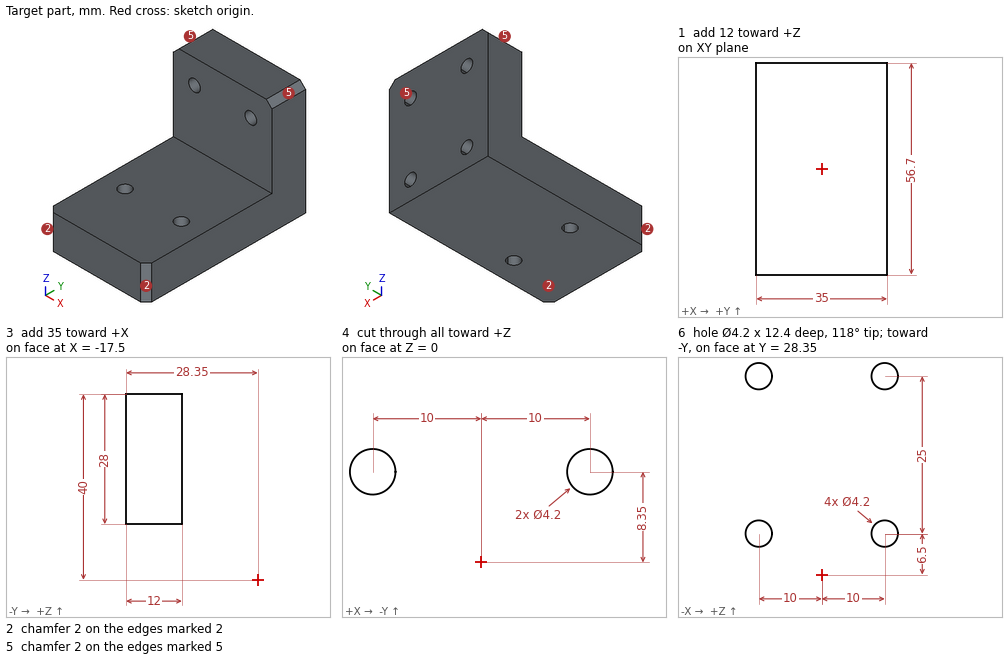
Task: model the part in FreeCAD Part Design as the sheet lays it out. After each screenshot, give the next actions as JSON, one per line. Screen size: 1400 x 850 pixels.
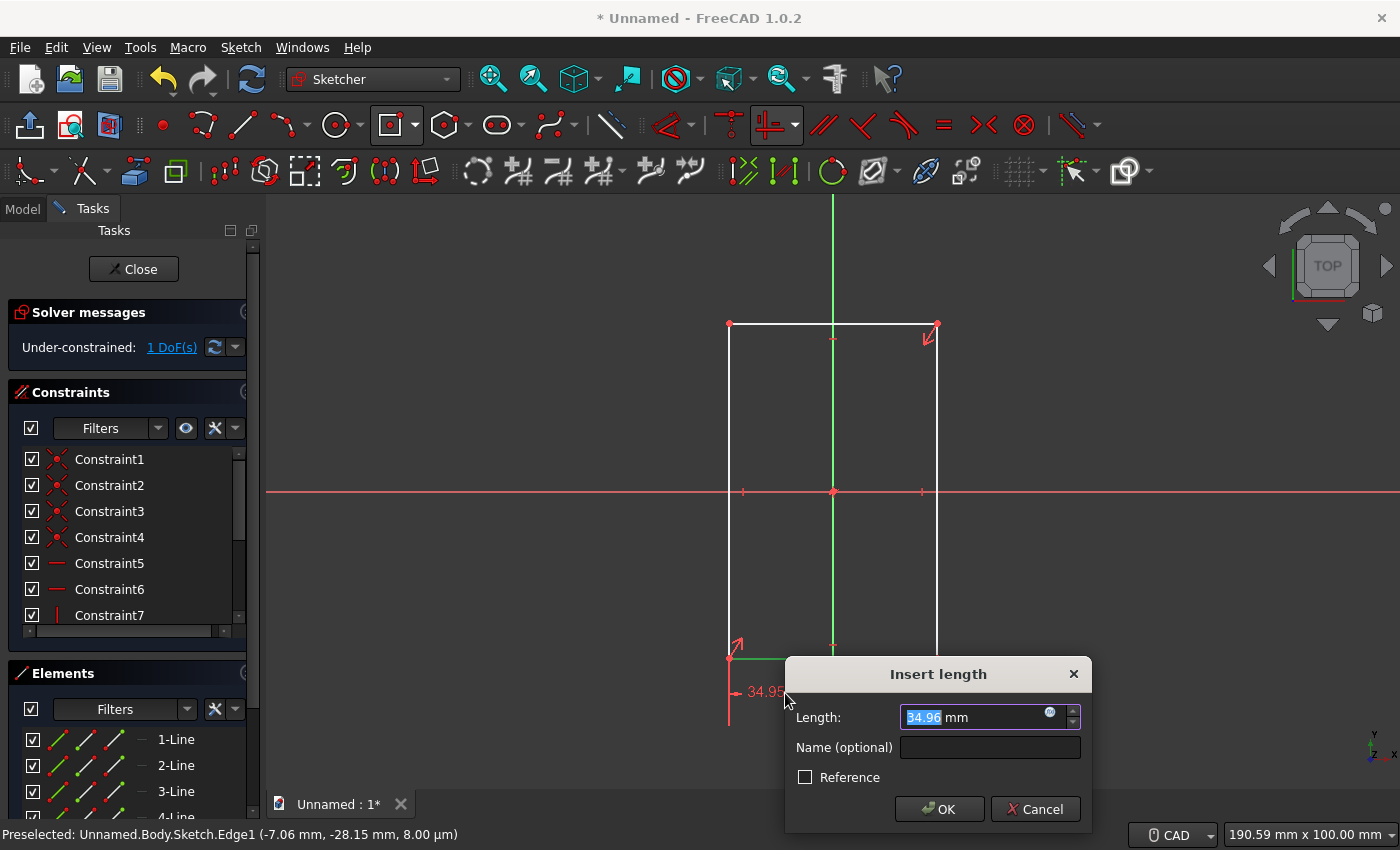
{"action": "type", "text": "35"}
{"action": "key", "text": "Return"}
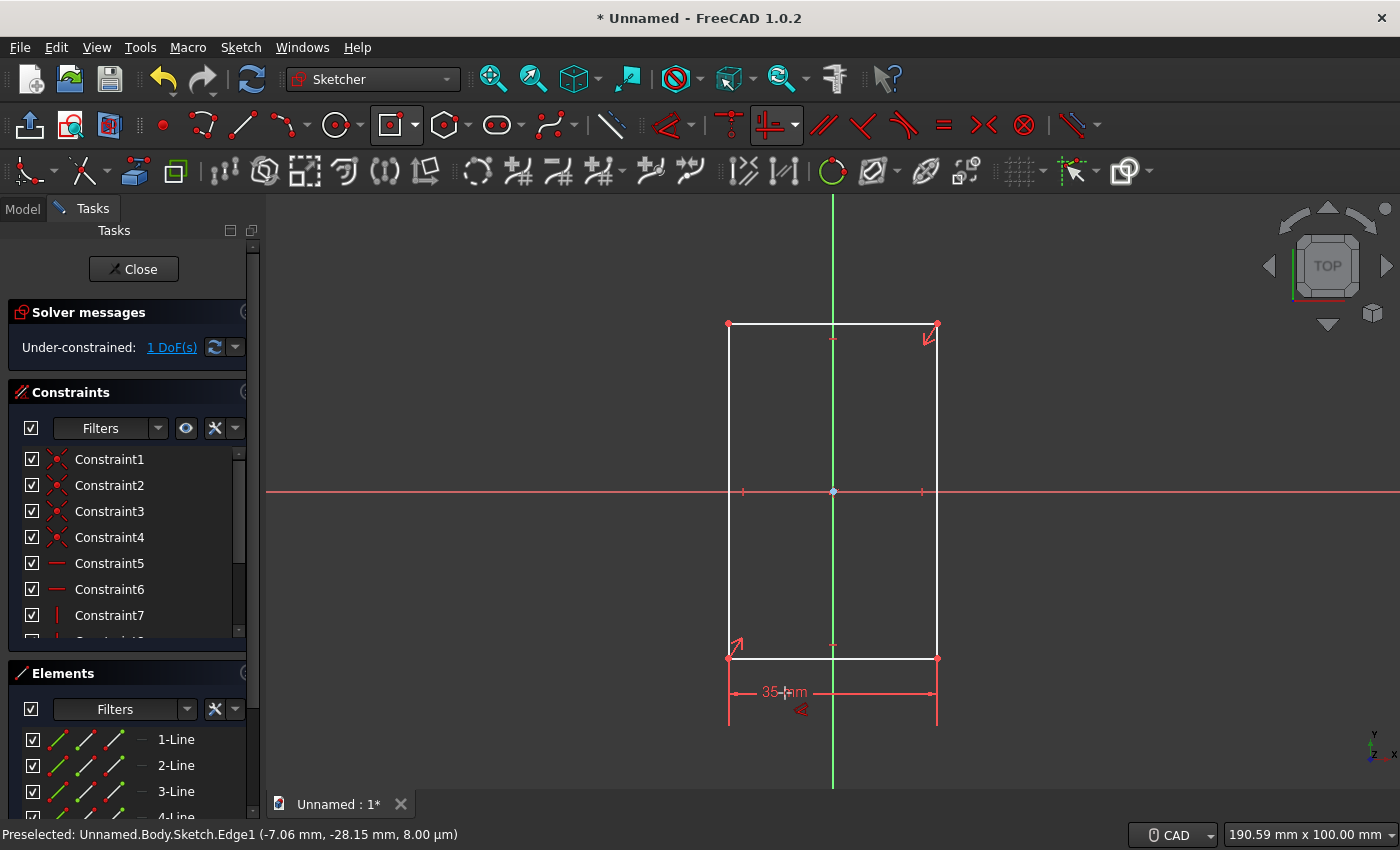
{"action": "left_click", "coordinate": [937, 559]}
{"action": "left_click", "coordinate": [971, 414]}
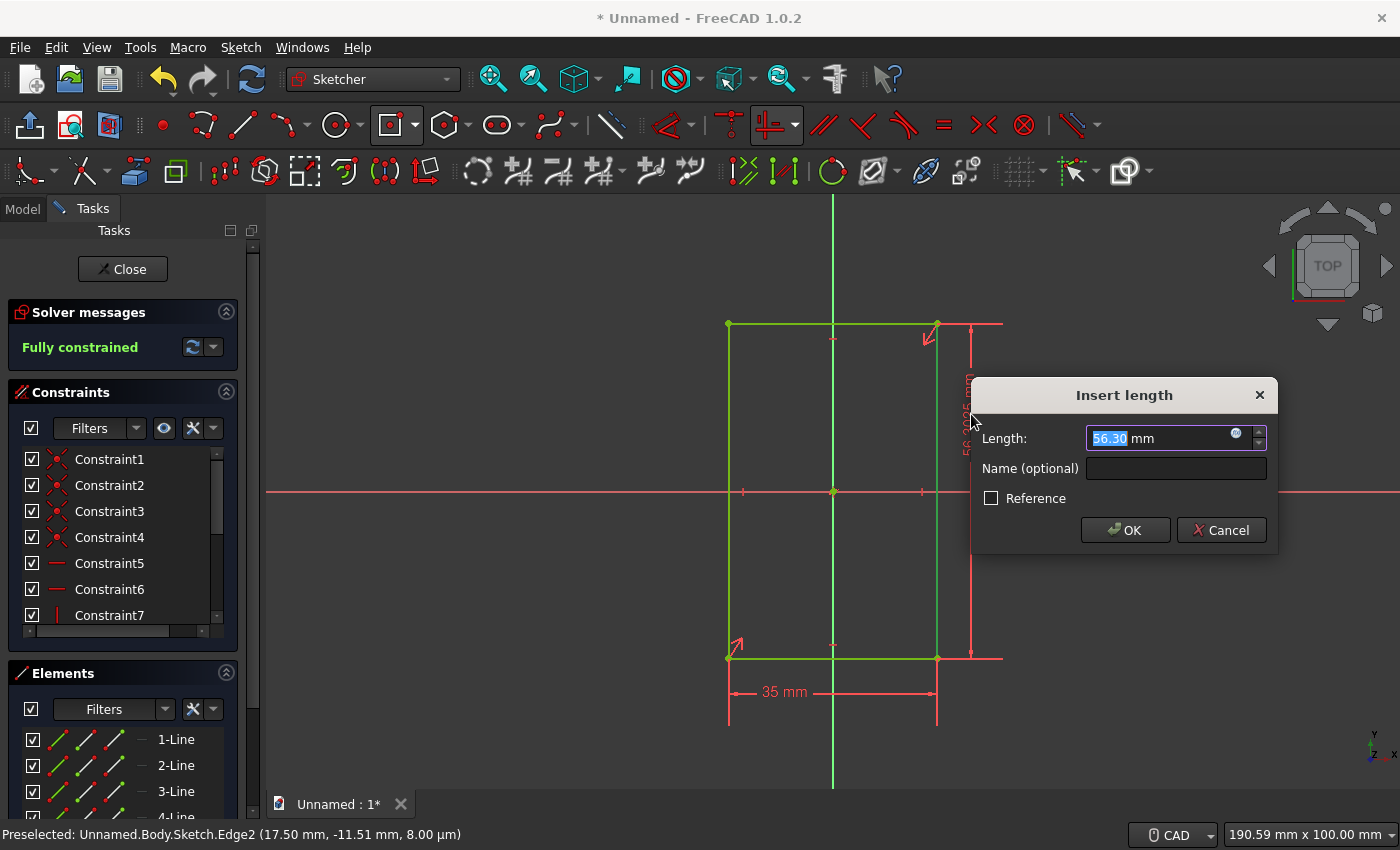
{"action": "type", "text": "56.7"}
{"action": "key", "text": "Return"}
{"action": "key", "text": "Escape"}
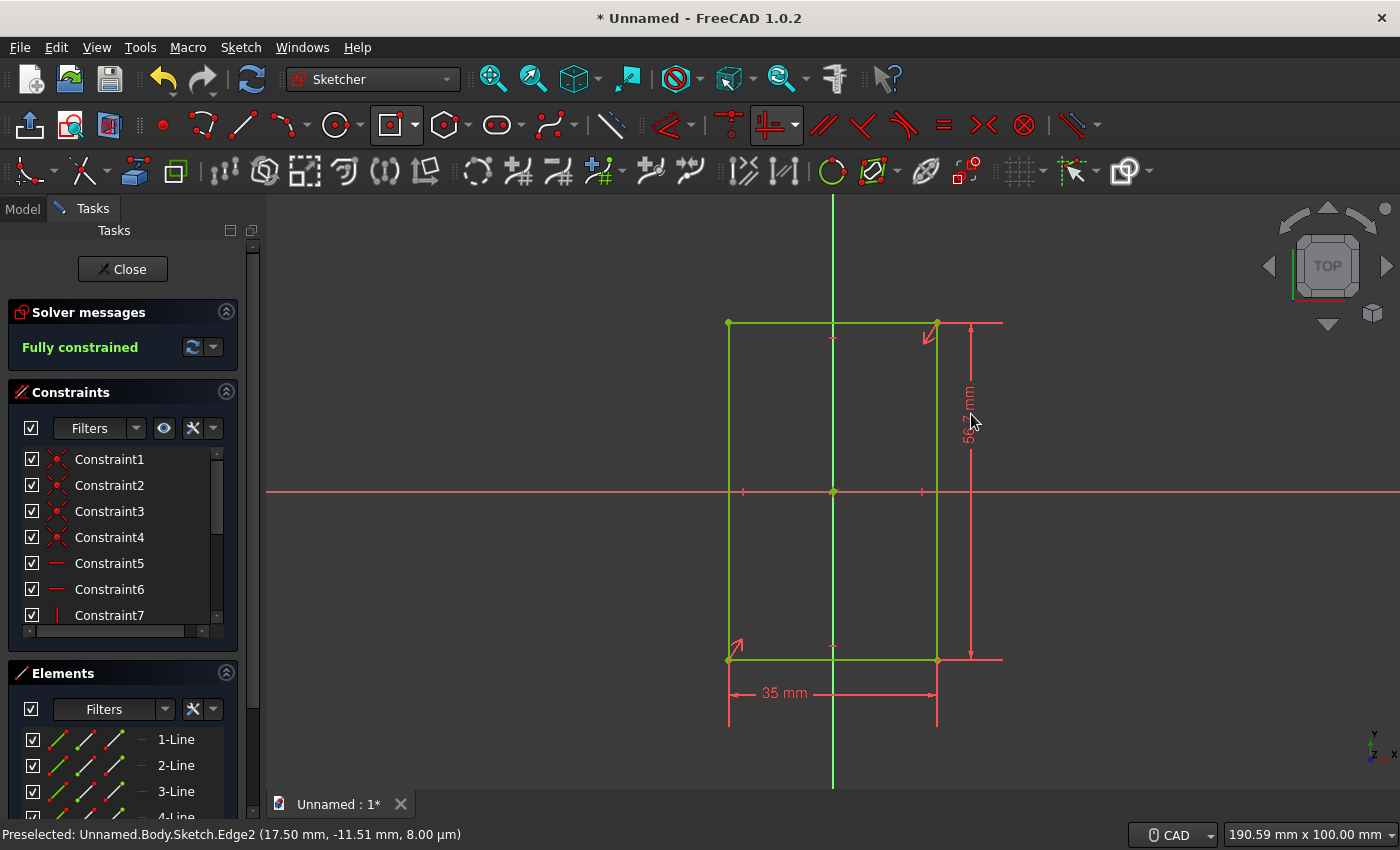
{"action": "left_click", "coordinate": [123, 269]}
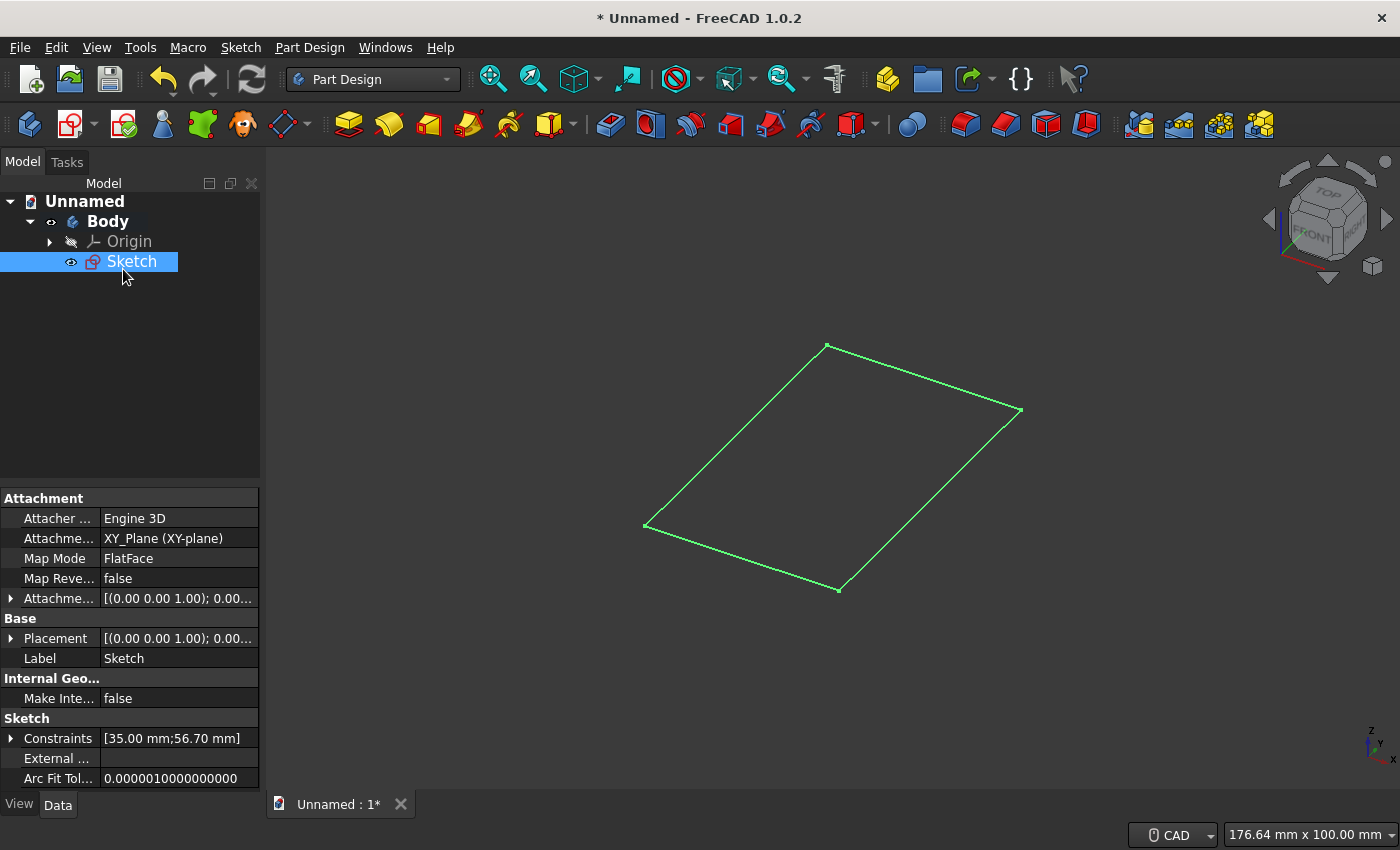
{"action": "left_click", "coordinate": [350, 124]}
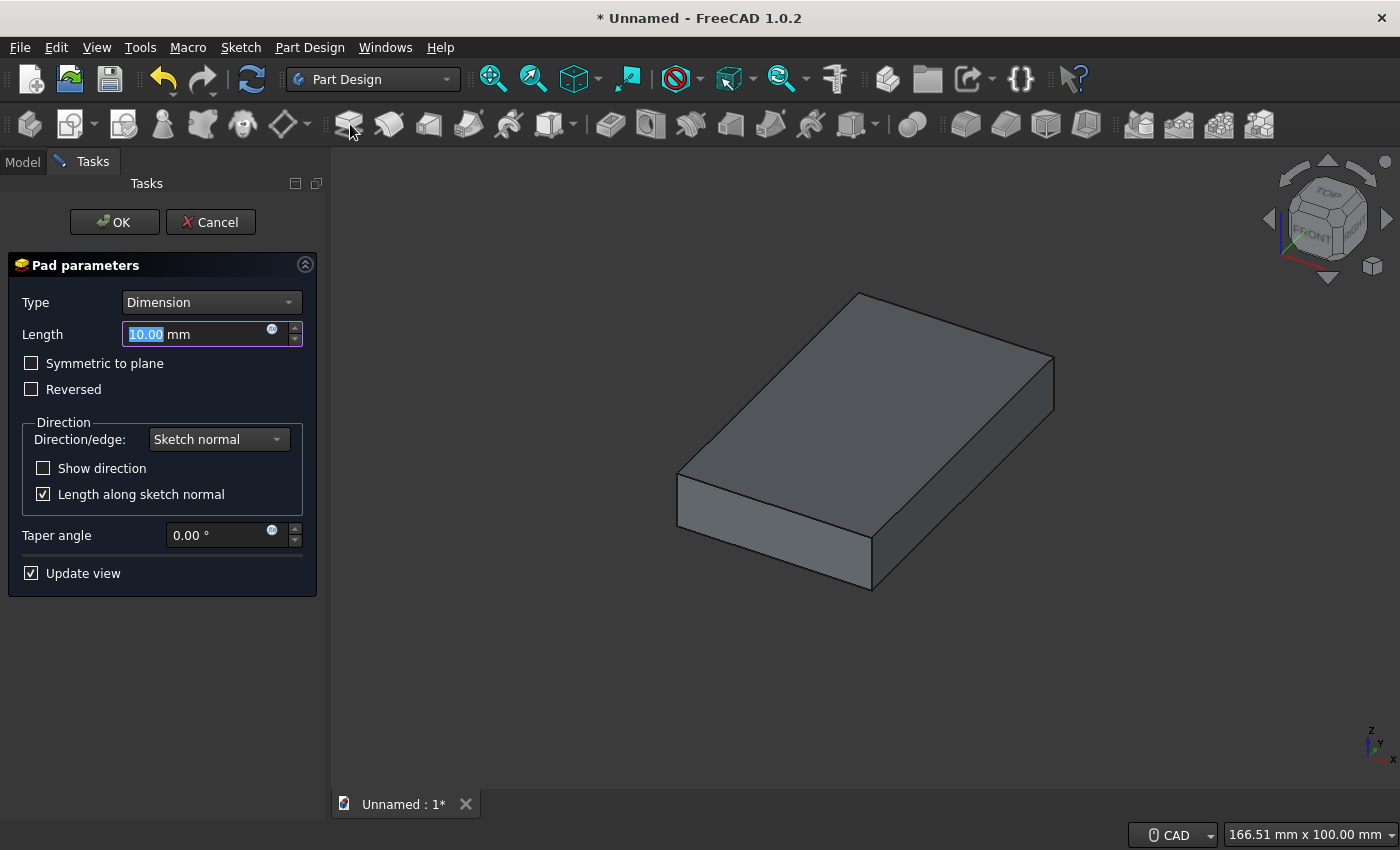
{"action": "type", "text": "12"}
{"action": "key", "text": "Tab"}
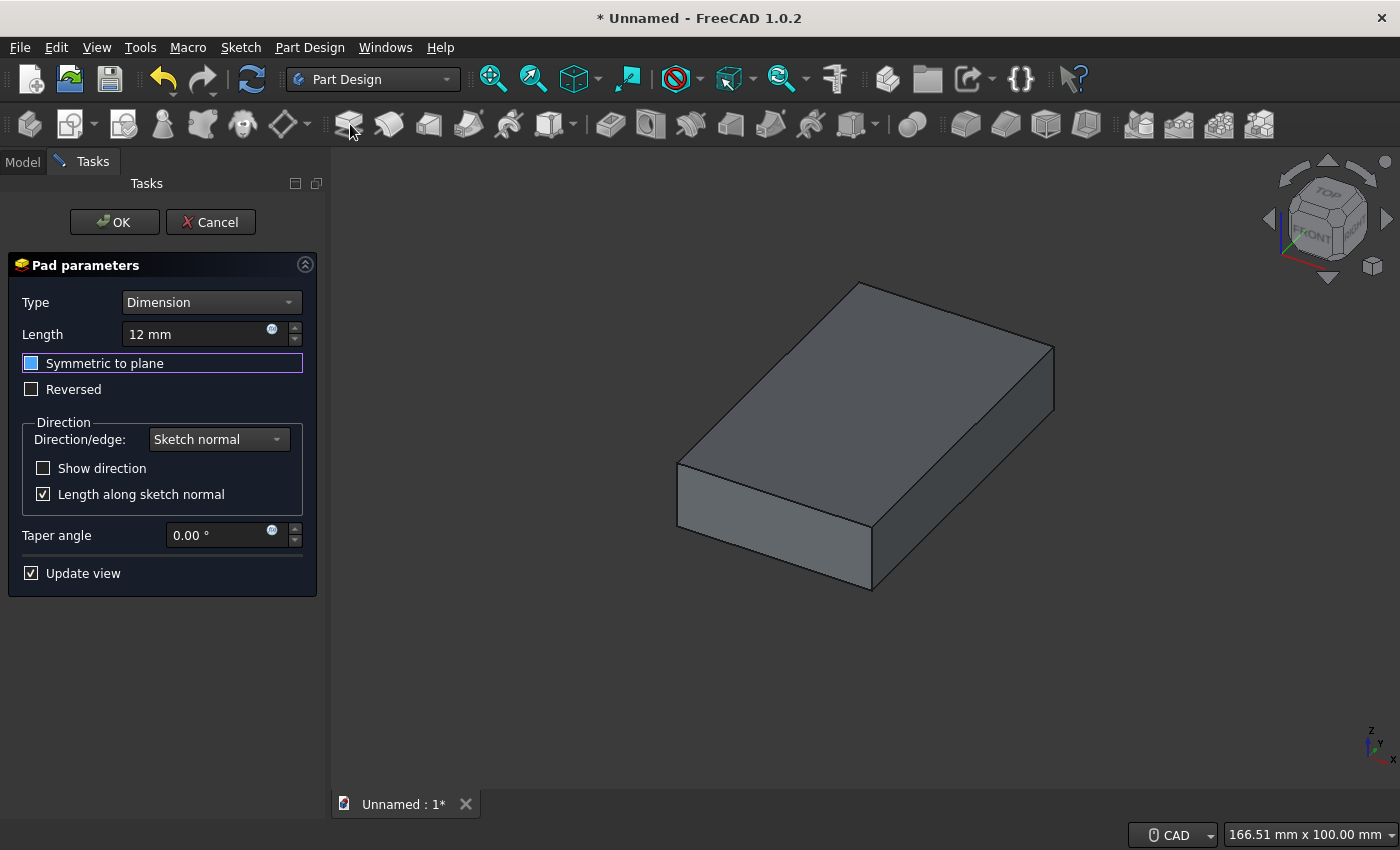
{"action": "left_click", "coordinate": [115, 222]}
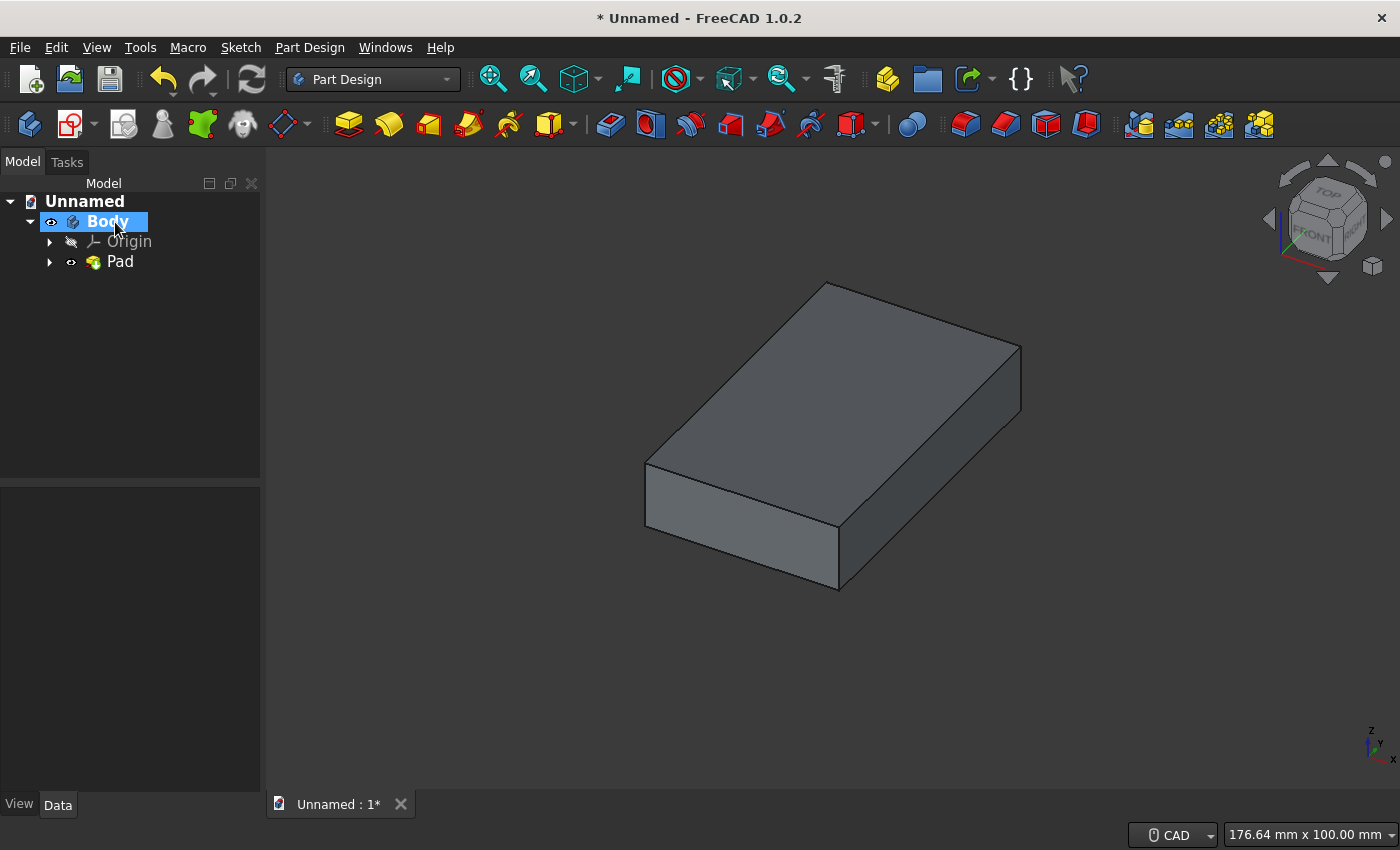
{"action": "left_click", "coordinate": [839, 558]}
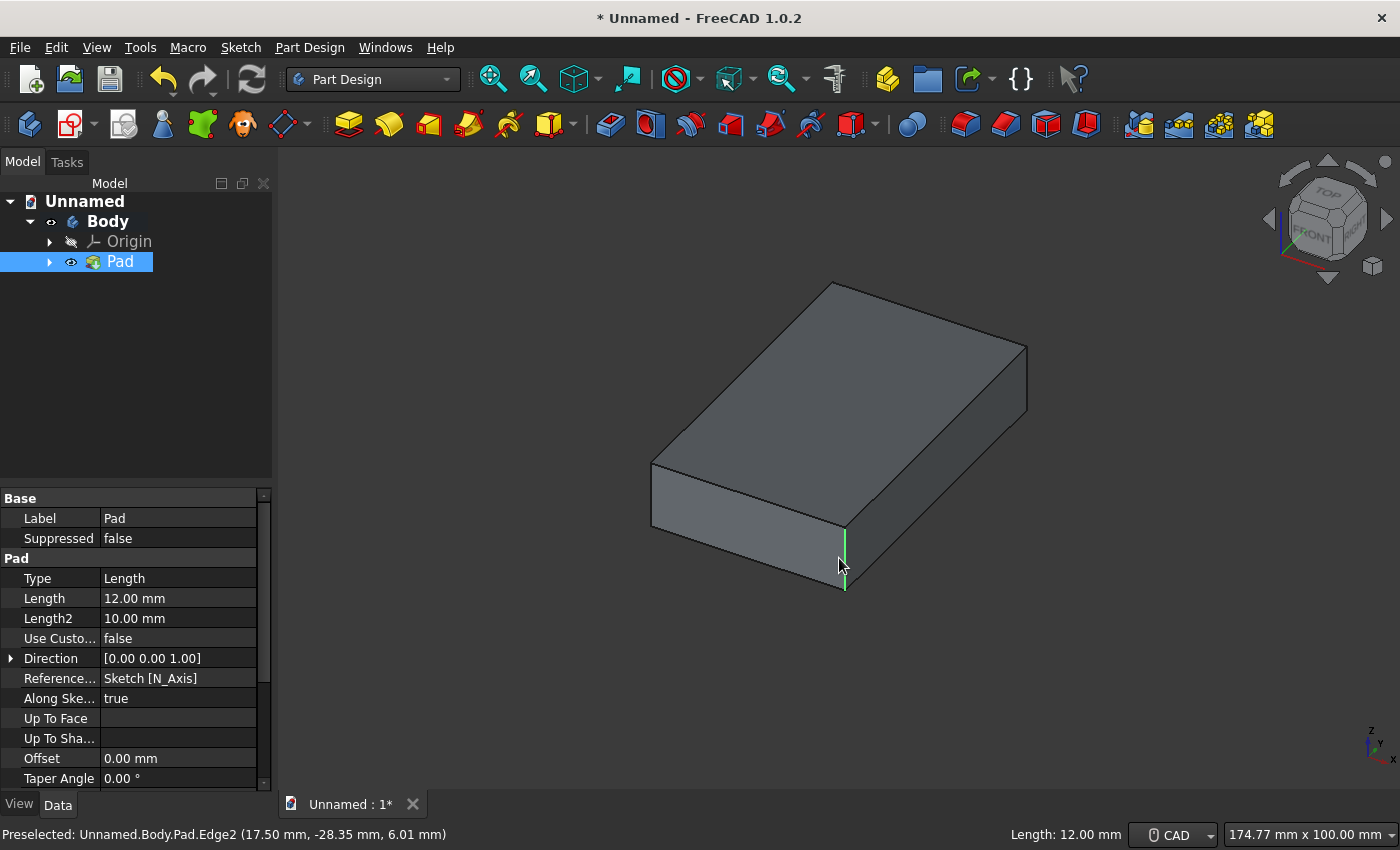
{"action": "key", "text": "0"}